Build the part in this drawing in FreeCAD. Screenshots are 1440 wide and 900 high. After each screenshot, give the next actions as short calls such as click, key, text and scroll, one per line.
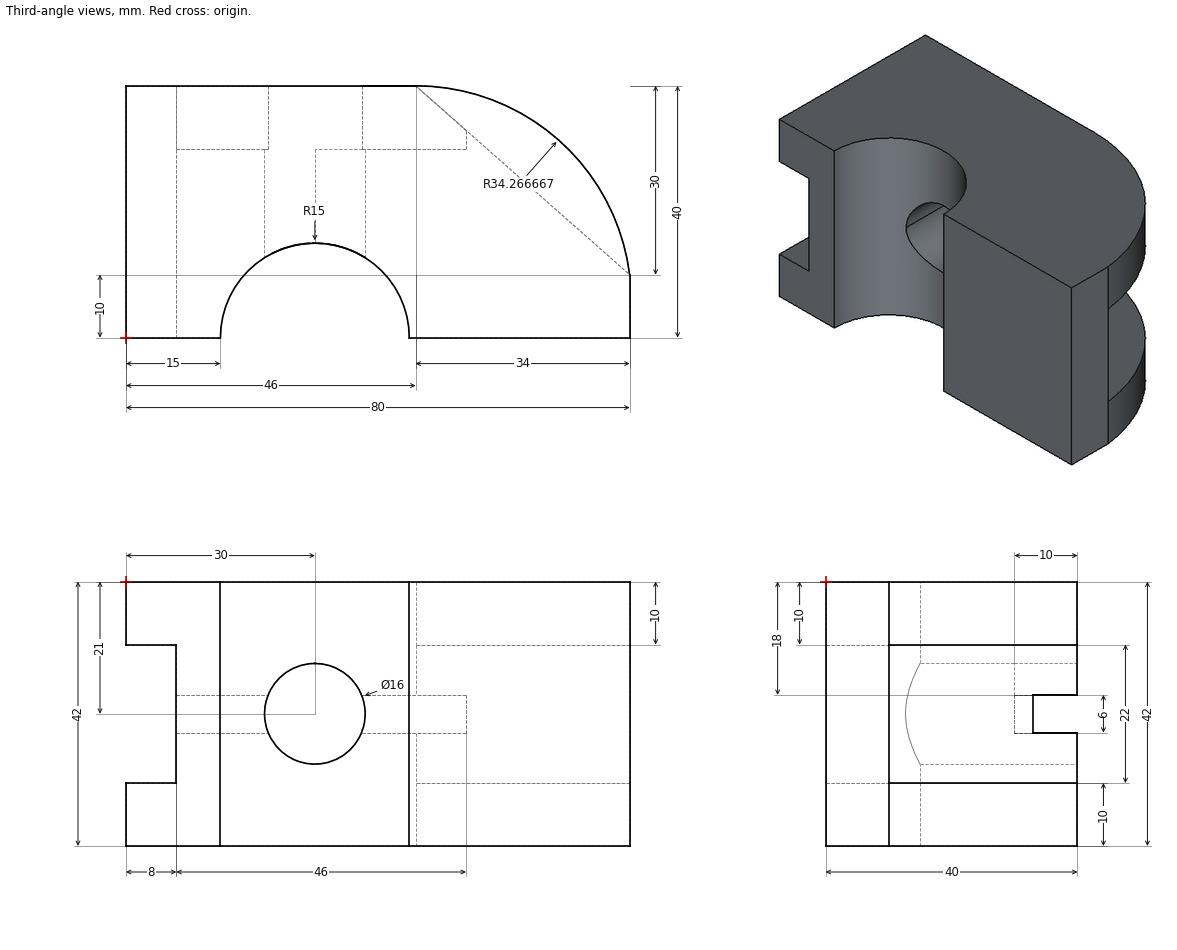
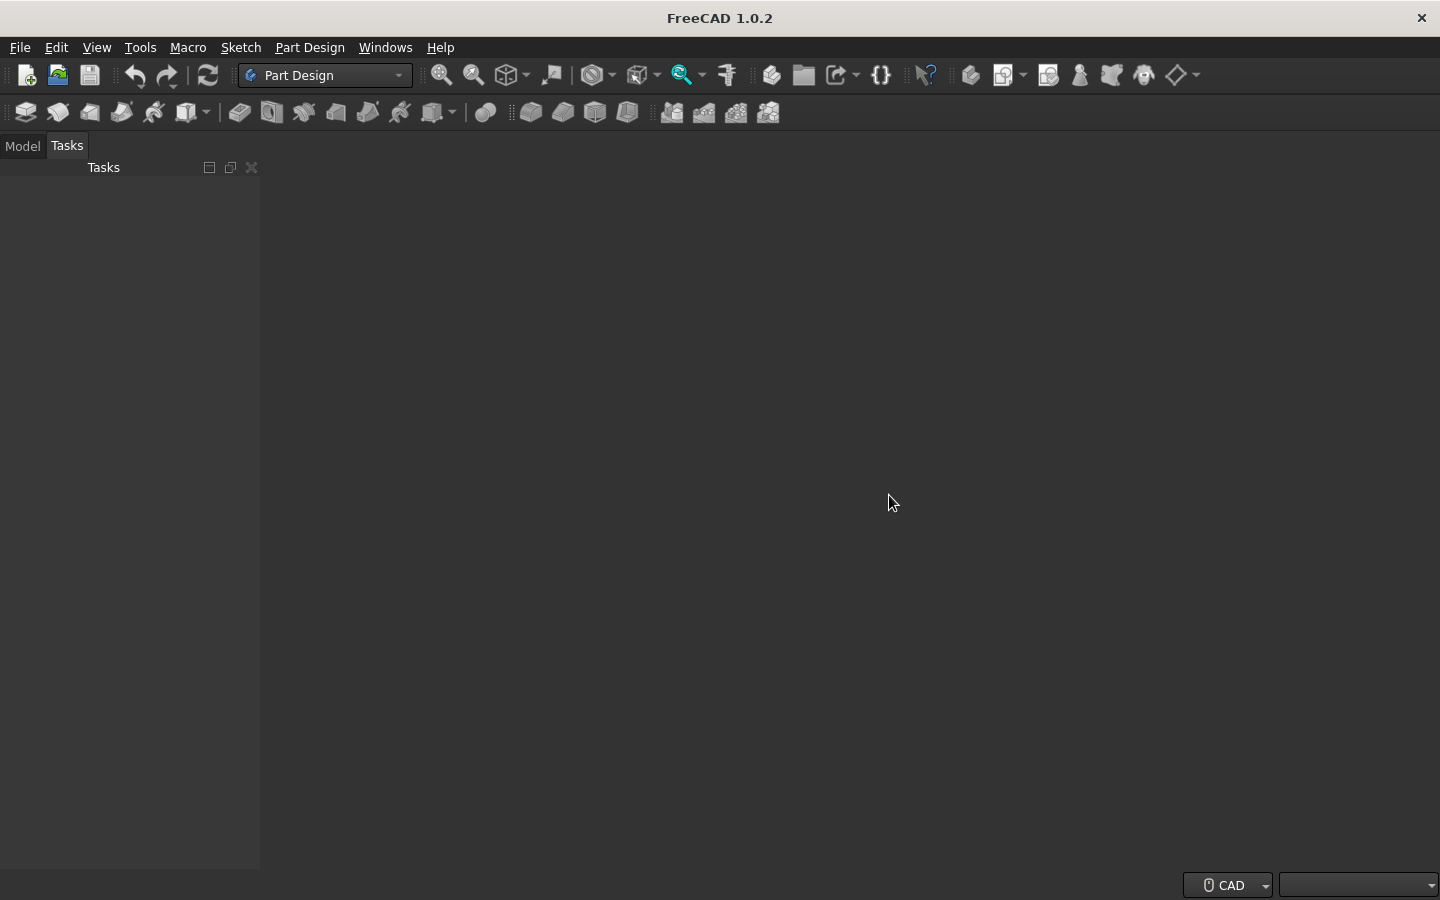
click(26, 76)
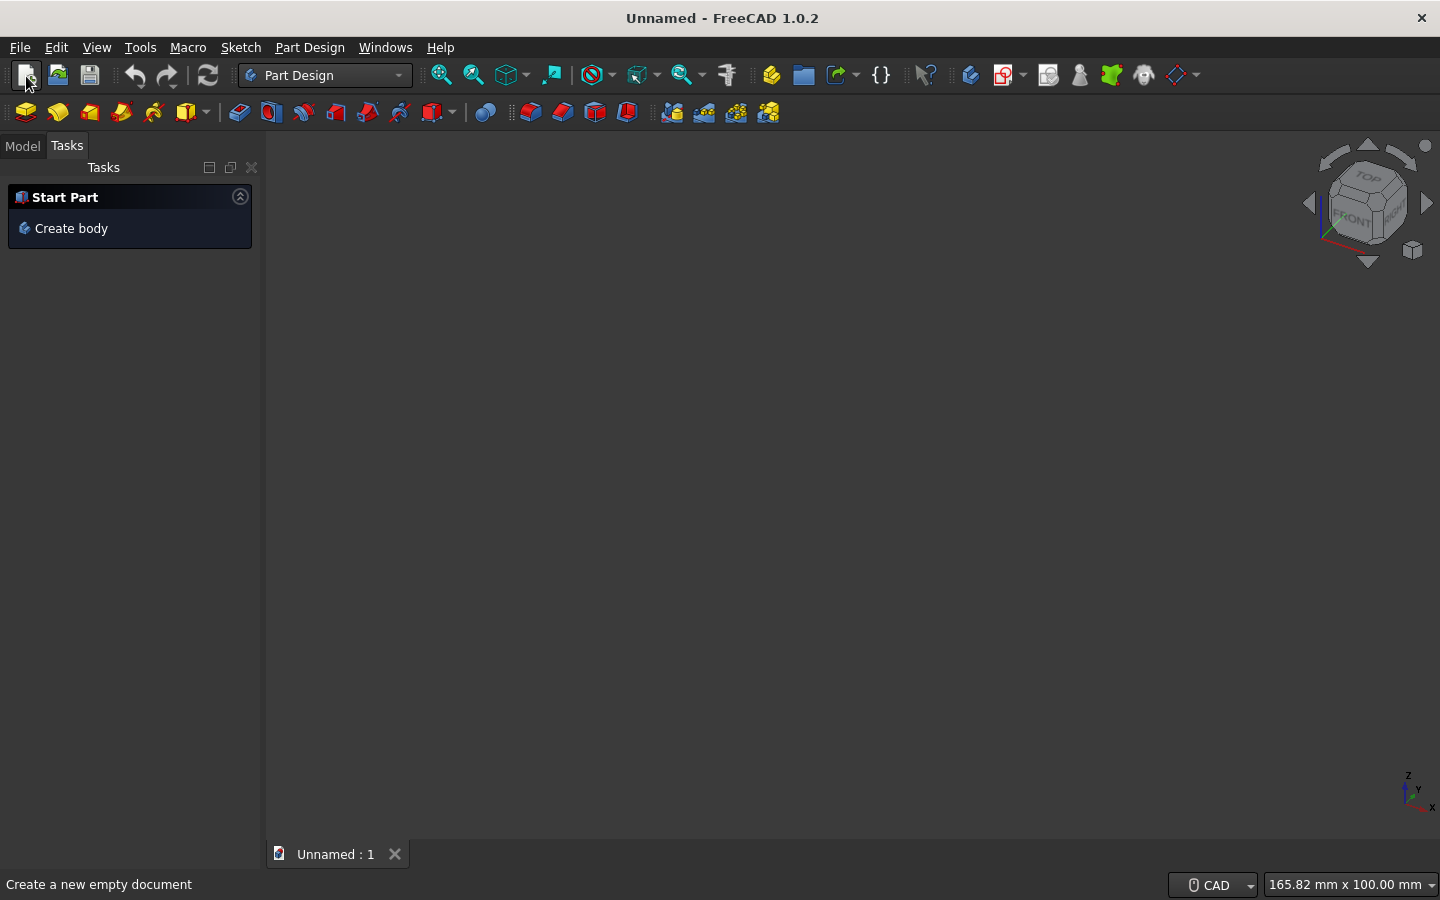
click(1004, 76)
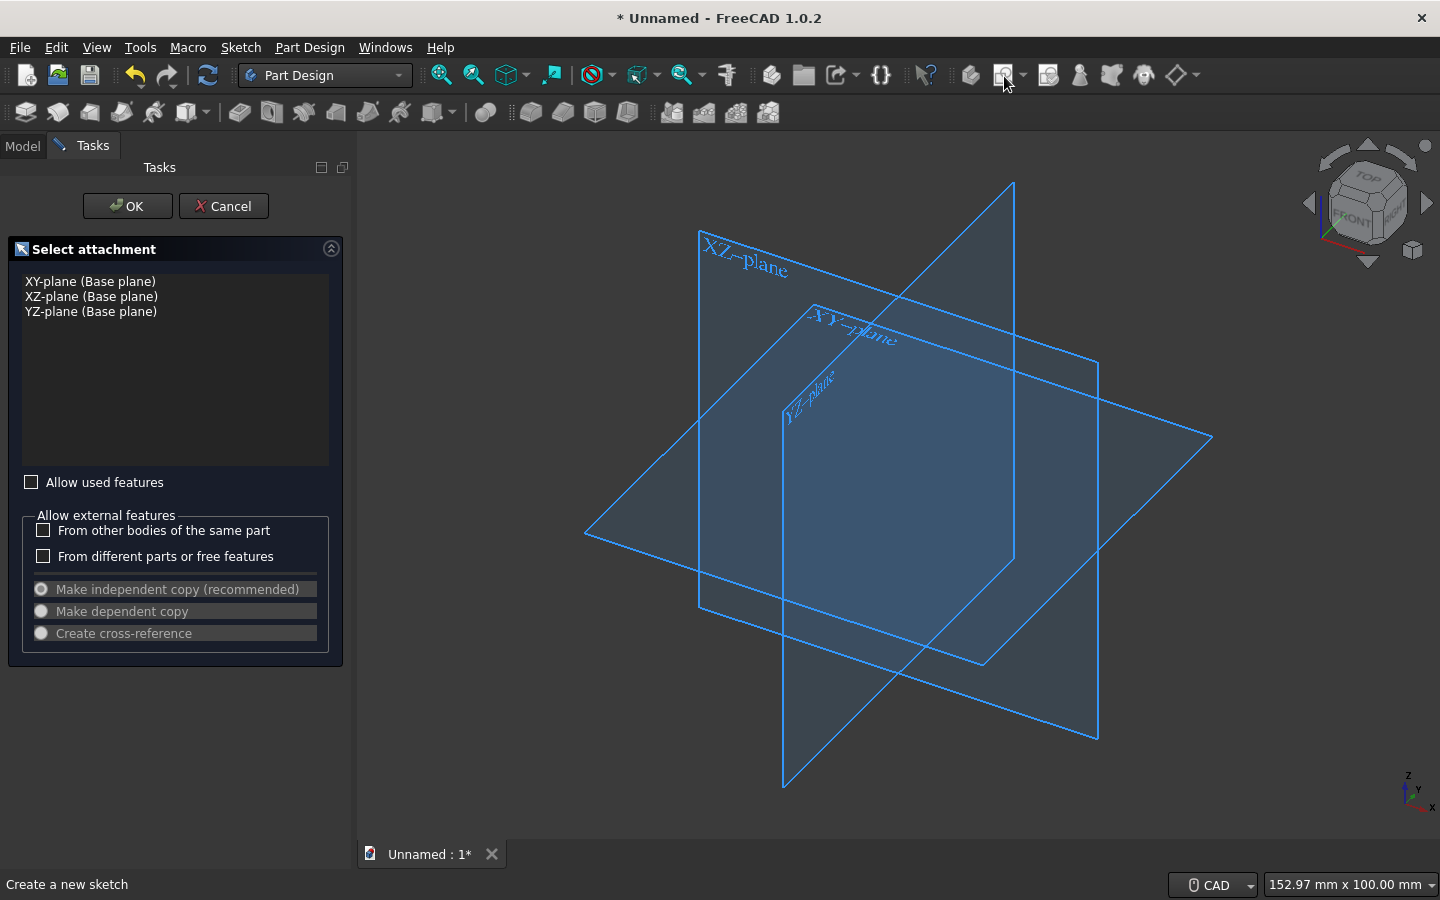
click(82, 282)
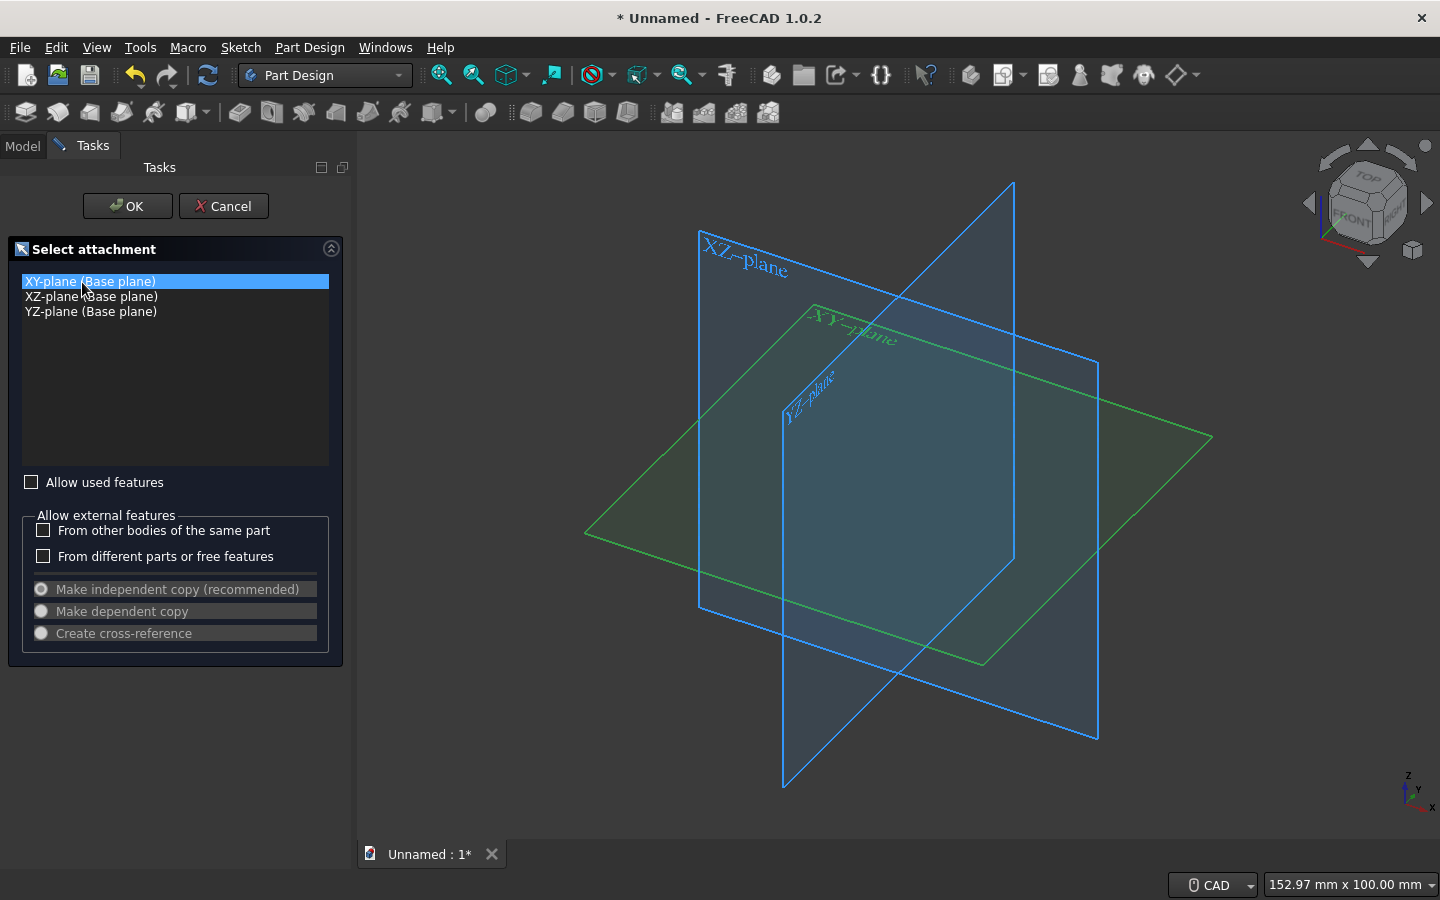
click(128, 206)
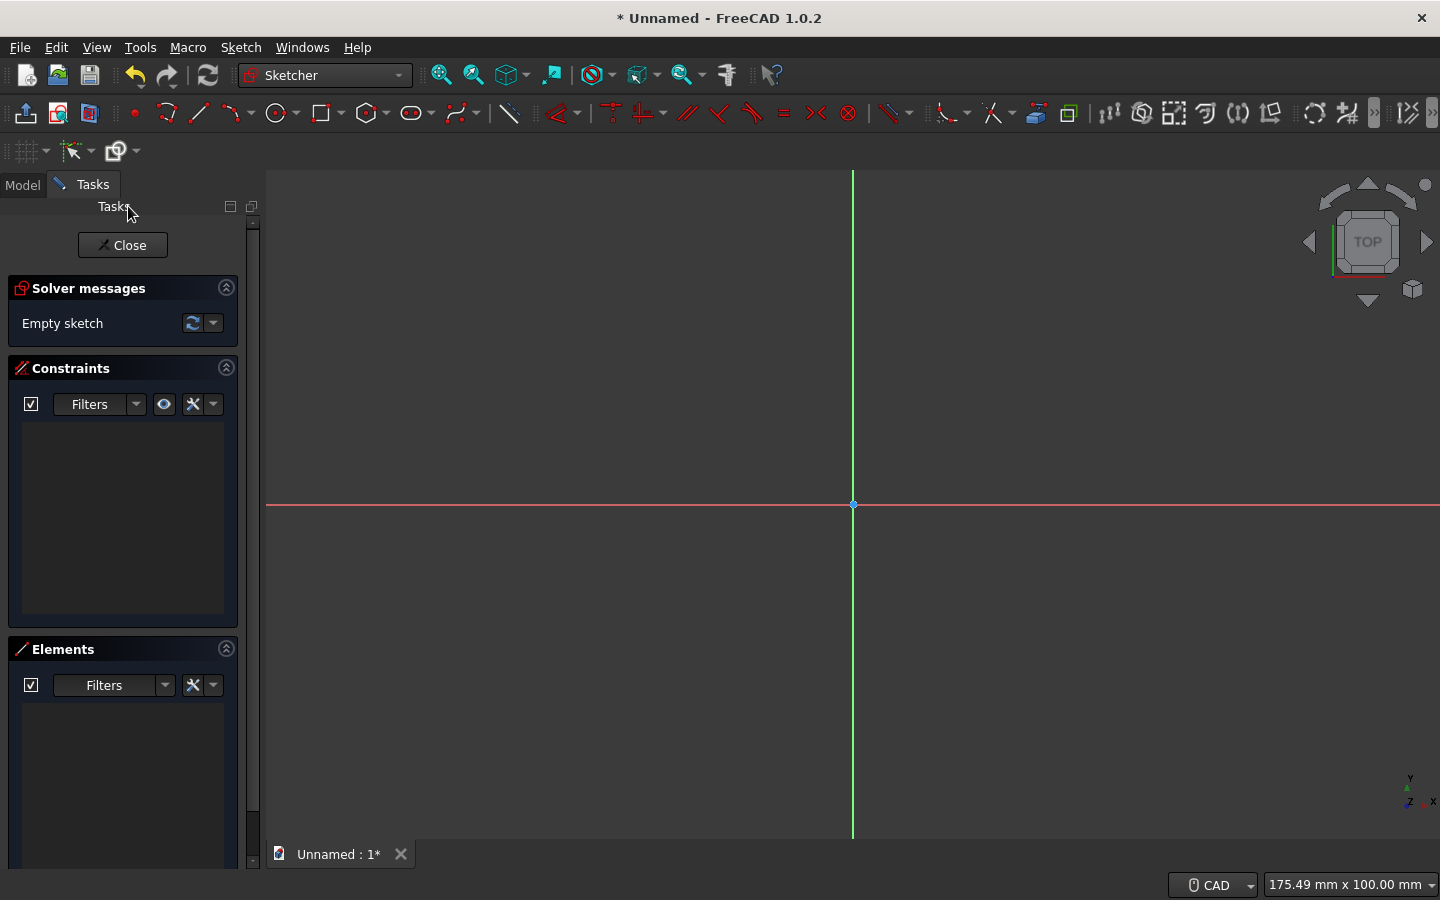
scroll(294, 811, down, 1)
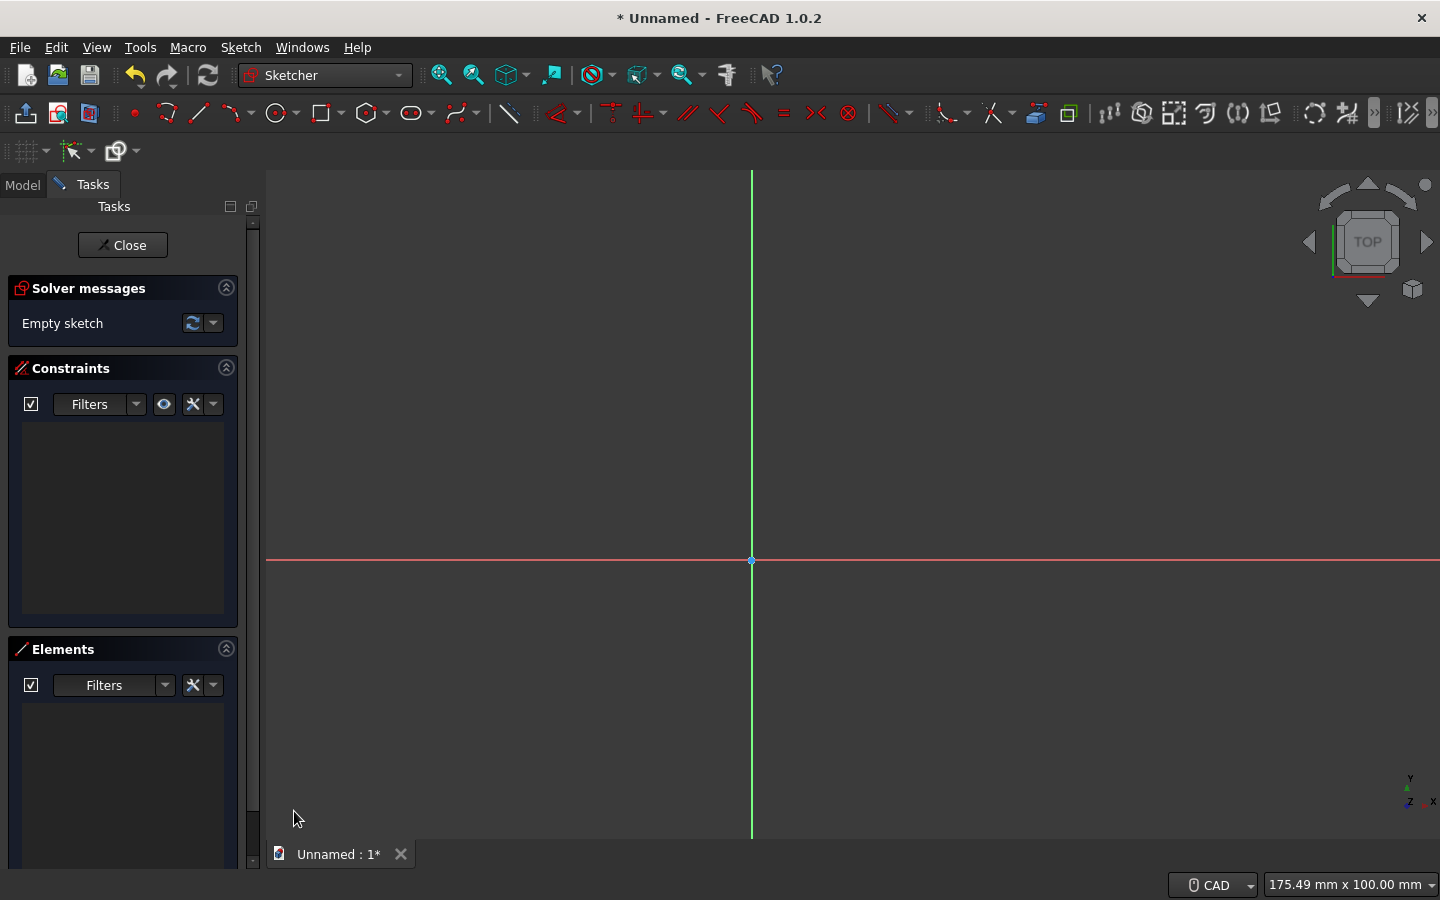
scroll(1275, 341, up, 2)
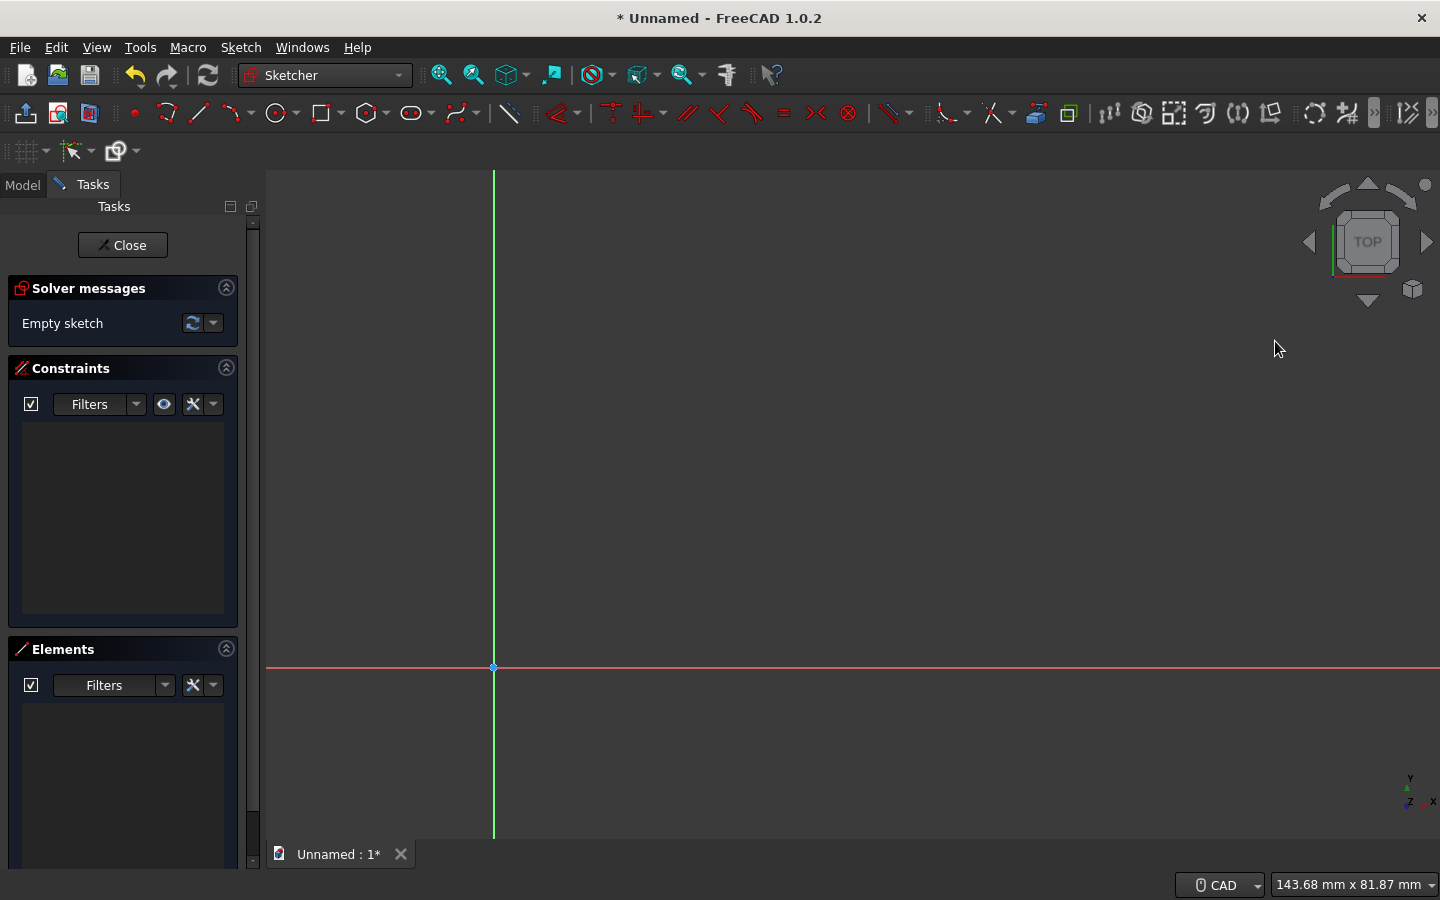
click(322, 114)